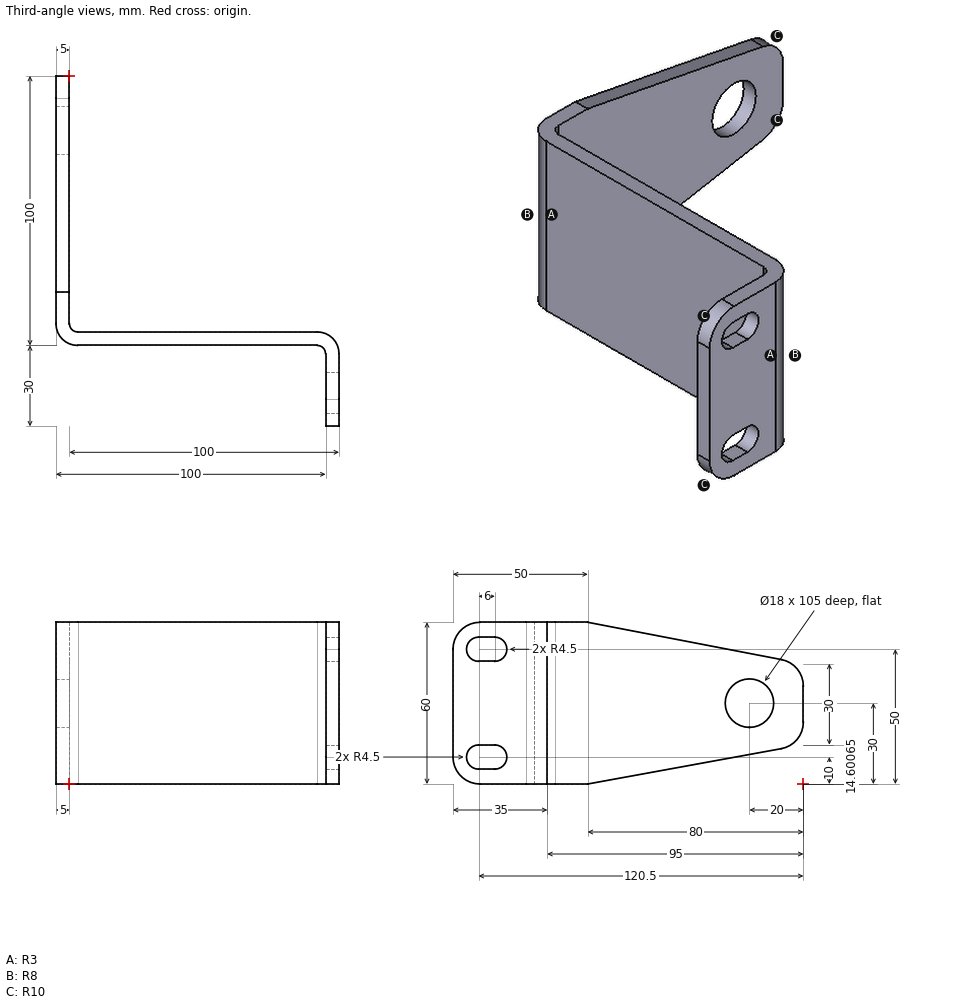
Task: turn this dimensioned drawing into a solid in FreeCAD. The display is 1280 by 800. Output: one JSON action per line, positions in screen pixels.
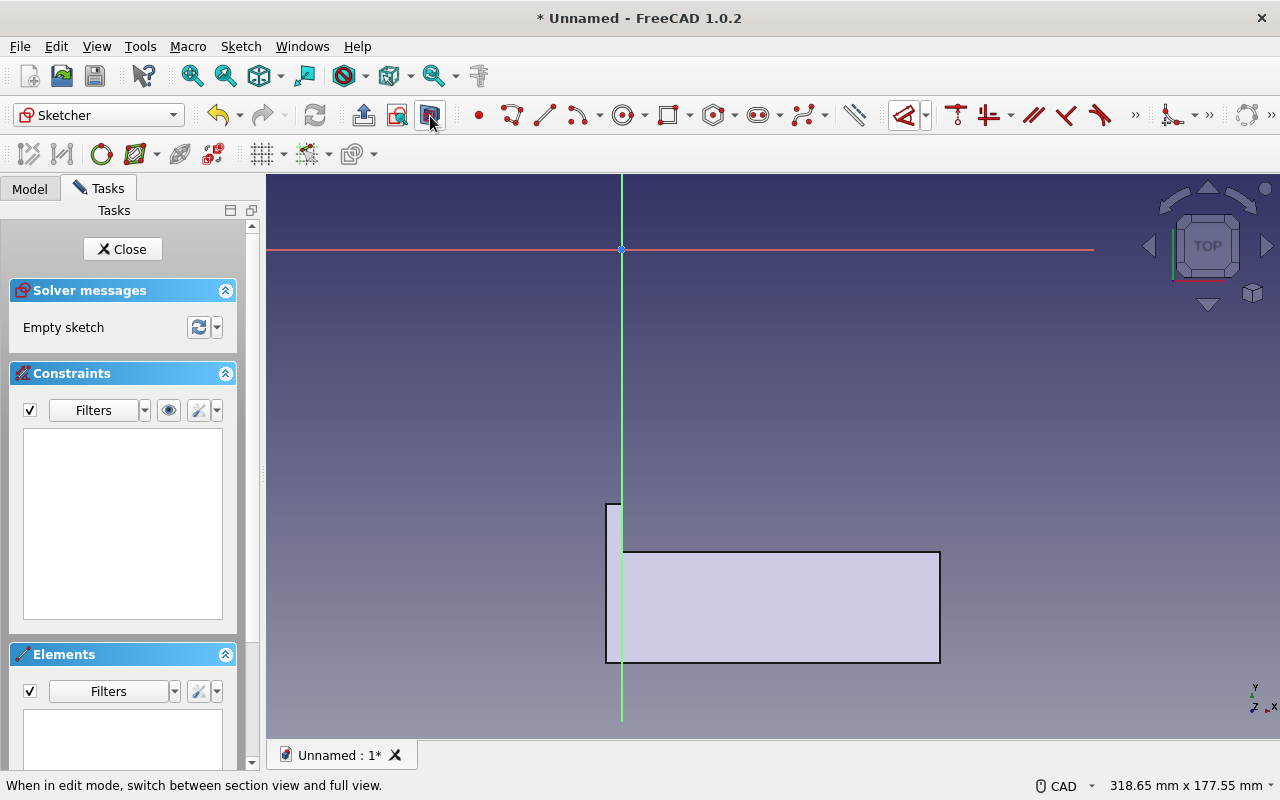
{"action": "left_click", "coordinate": [668, 116]}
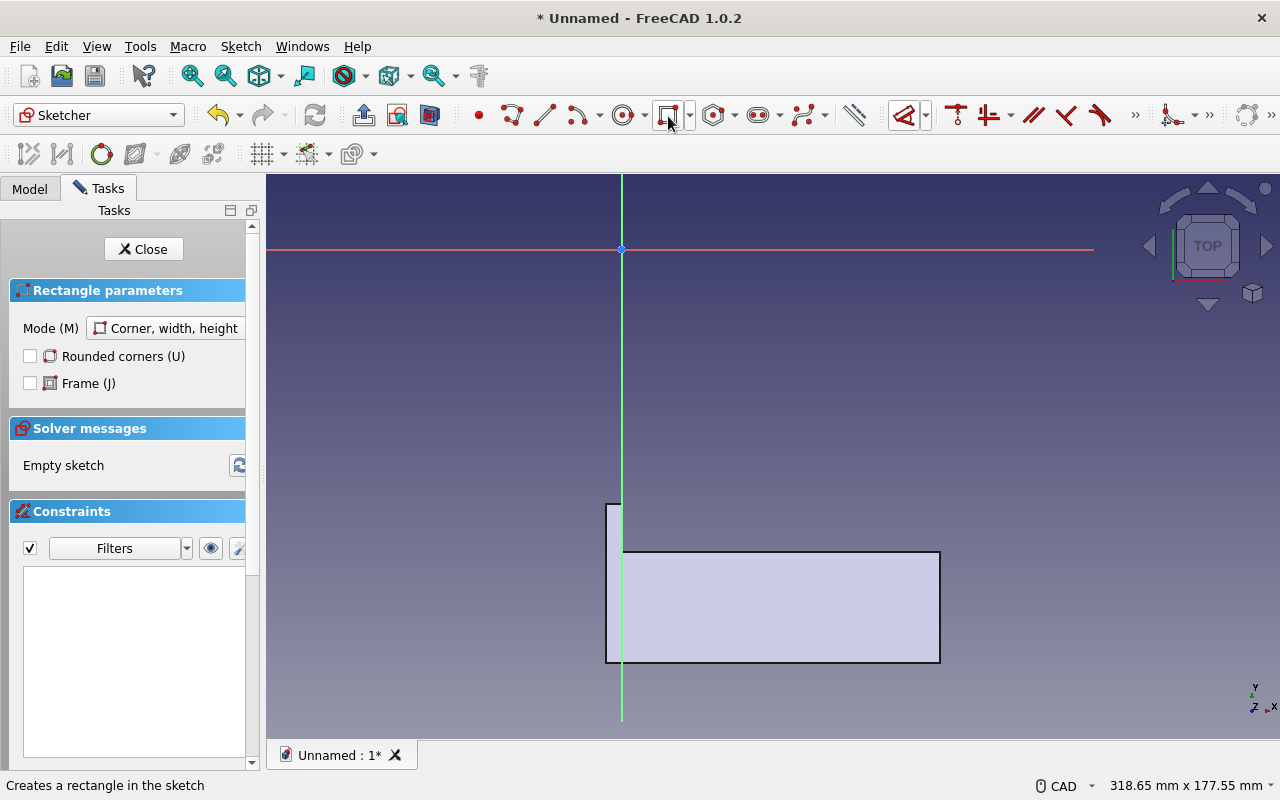
{"action": "left_click", "coordinate": [606, 568]}
{"action": "left_click", "coordinate": [924, 663]}
{"action": "key", "text": "Escape"}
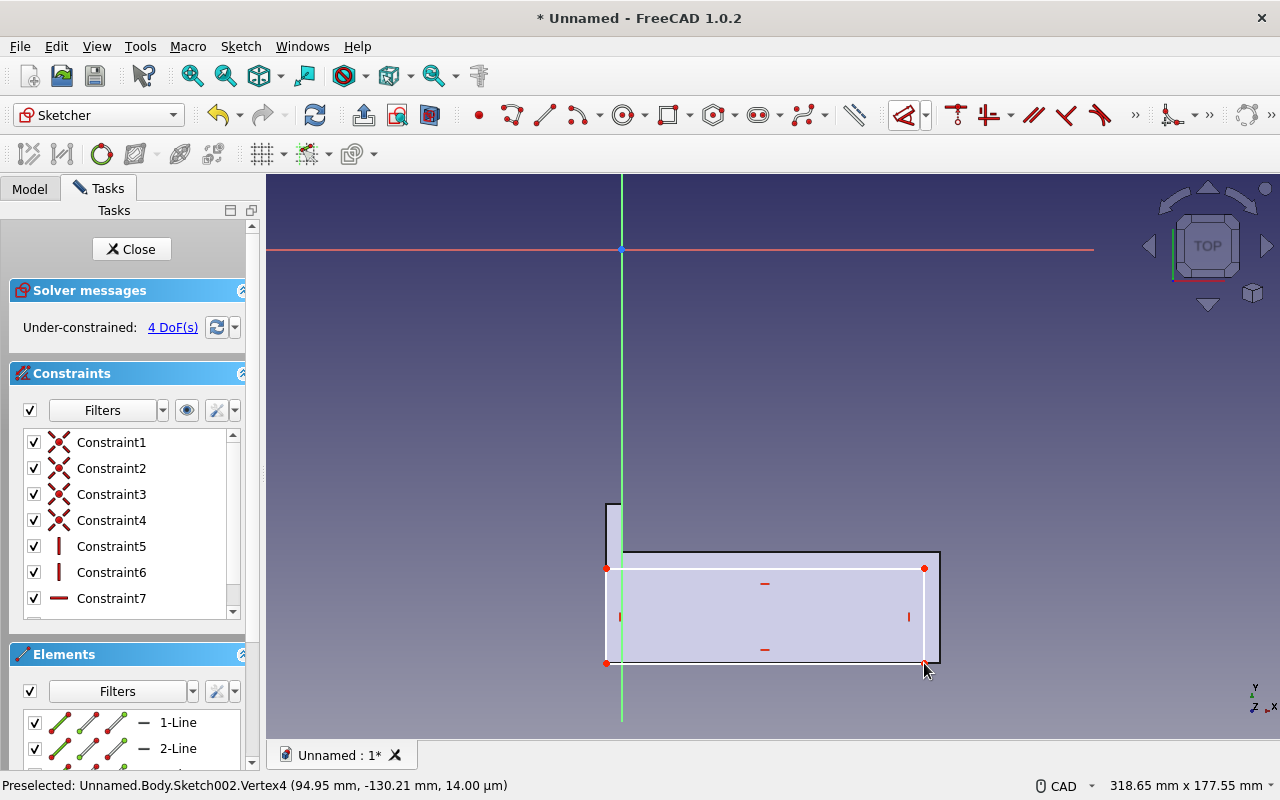
{"action": "left_click", "coordinate": [606, 597]}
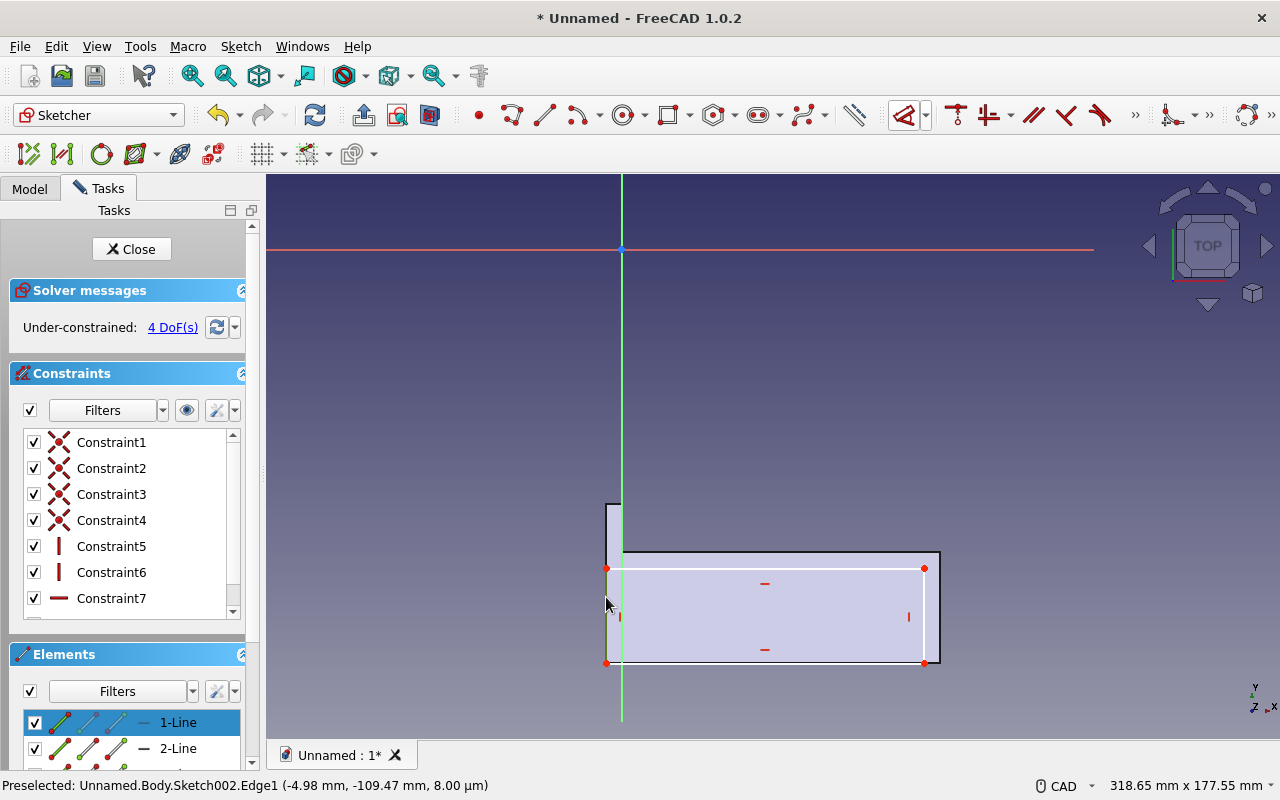
{"action": "key", "text": "i"}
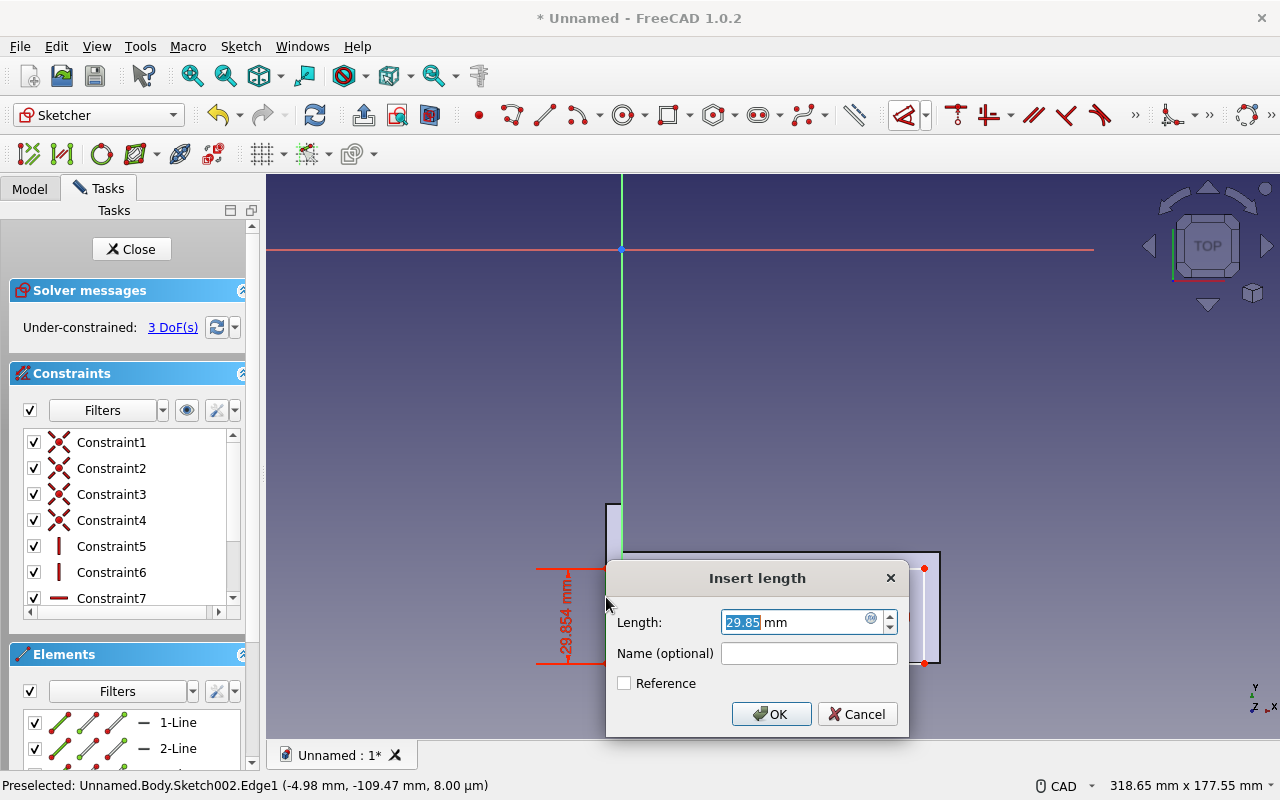
{"action": "type", "text": "30"}
{"action": "key", "text": "Return"}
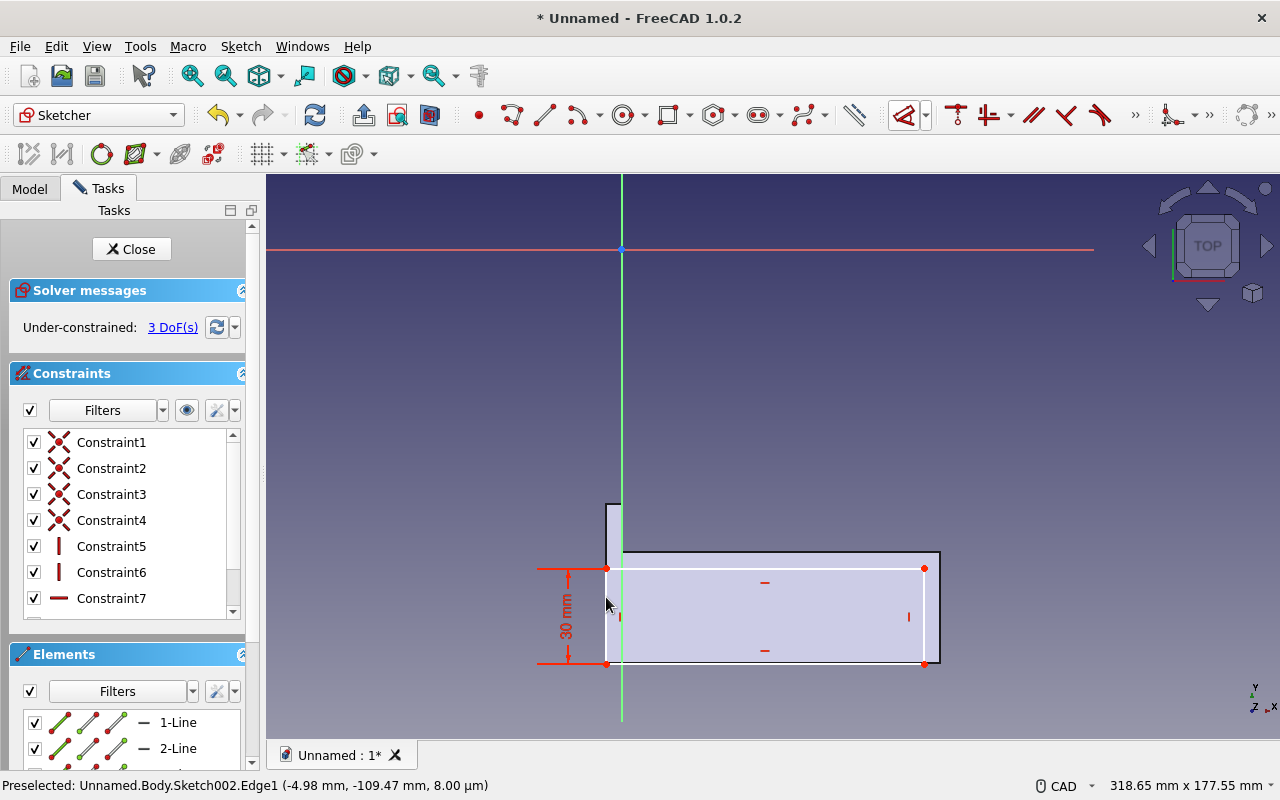
{"action": "scroll", "coordinate": [606, 569], "scroll_direction": "up", "scroll_amount": 5}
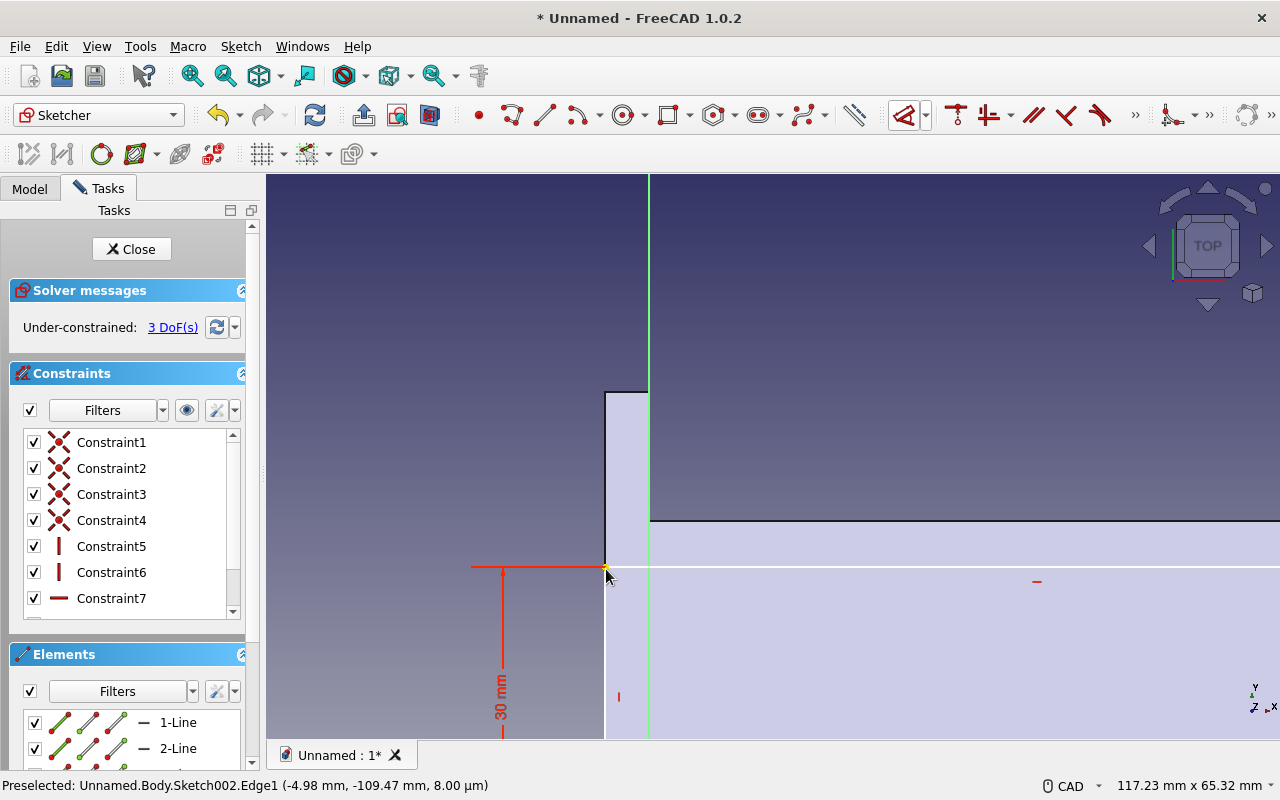
{"action": "left_click", "coordinate": [605, 567]}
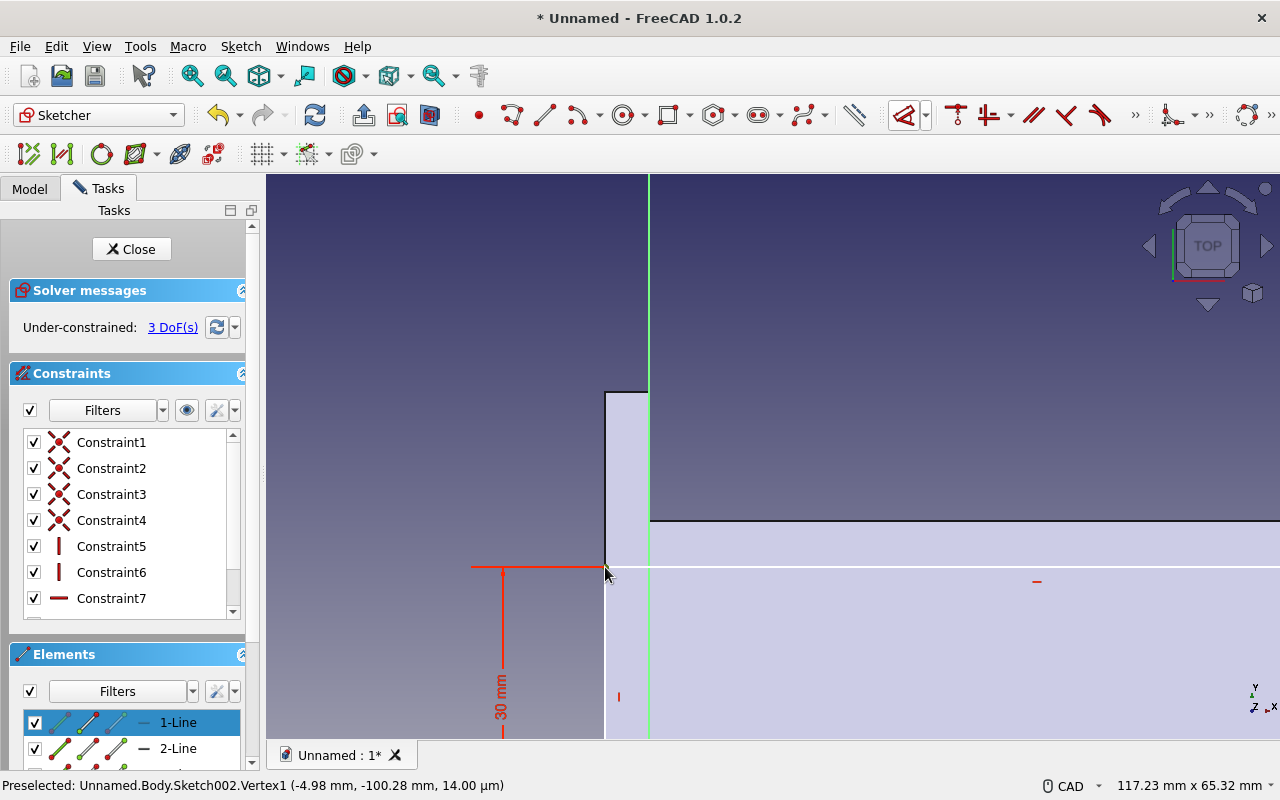
{"action": "key", "text": "l"}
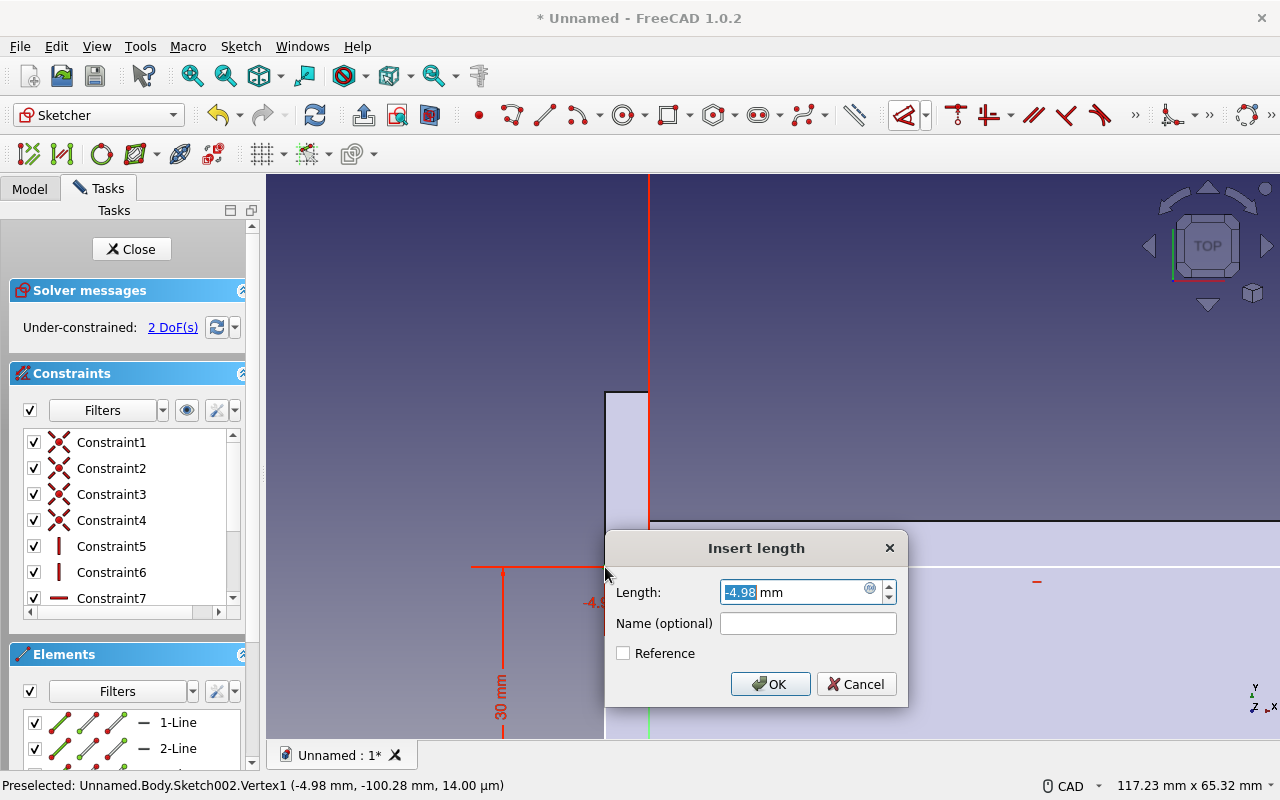
{"action": "type", "text": "-5"}
{"action": "key", "text": "Return"}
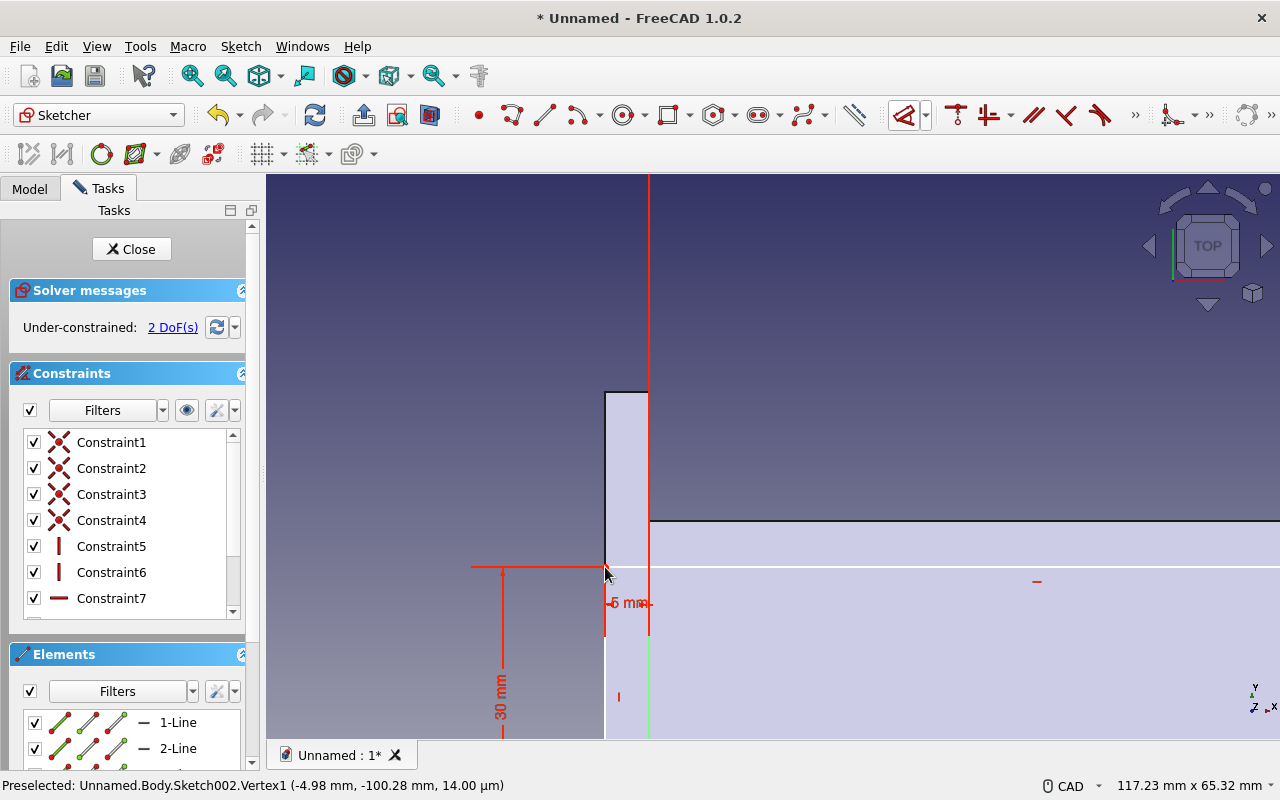
{"action": "scroll", "coordinate": [561, 540], "scroll_direction": "down", "scroll_amount": 6}